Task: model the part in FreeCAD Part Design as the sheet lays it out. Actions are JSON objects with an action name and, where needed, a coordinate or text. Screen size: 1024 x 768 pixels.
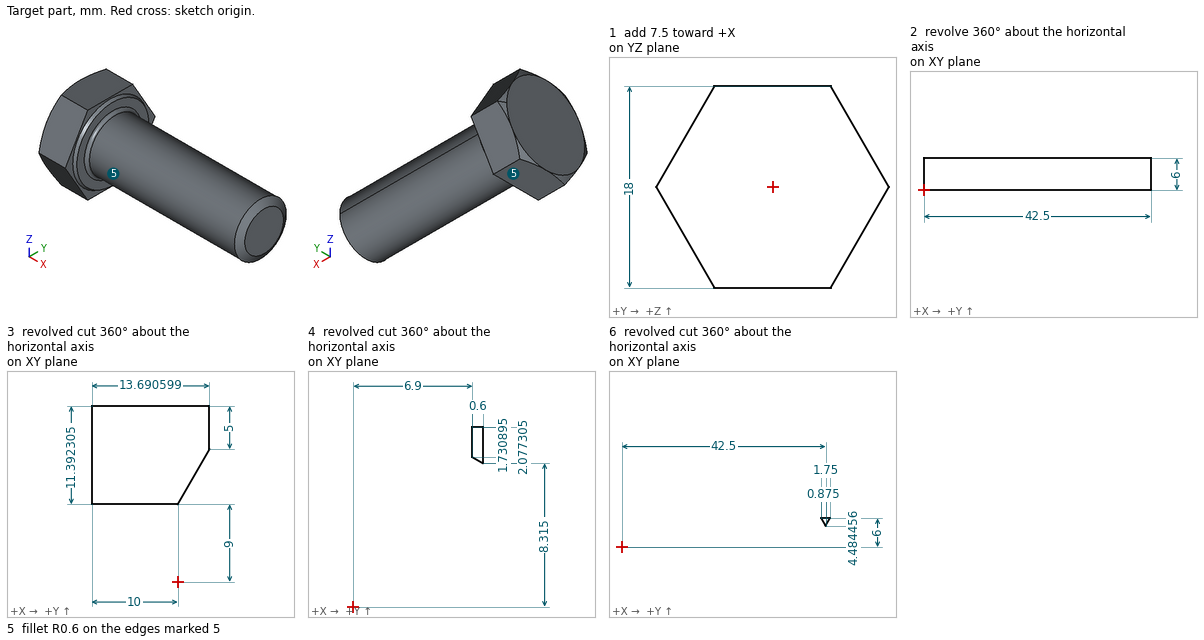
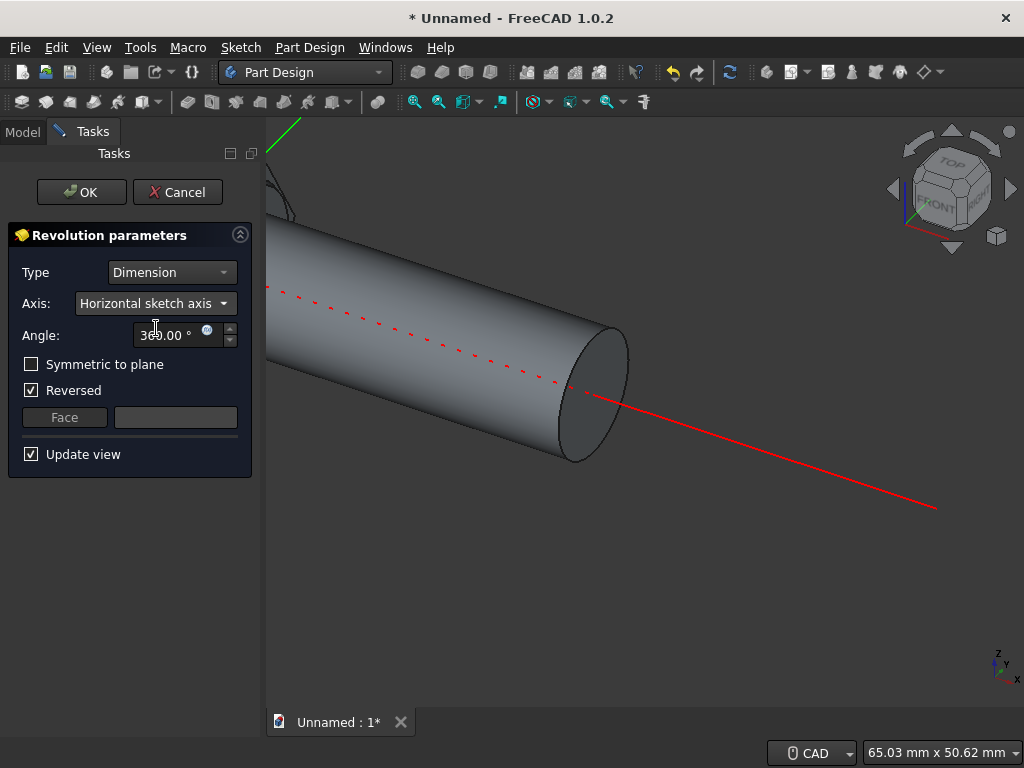
{"action": "left_click", "coordinate": [82, 192]}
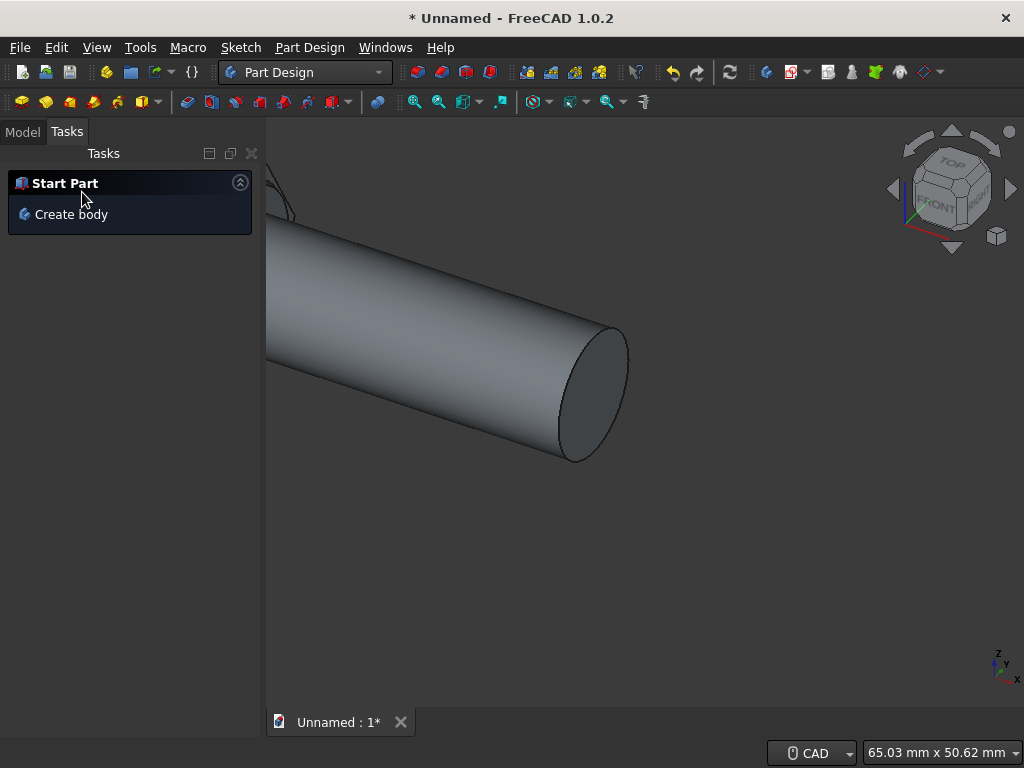
{"action": "left_click", "coordinate": [416, 102]}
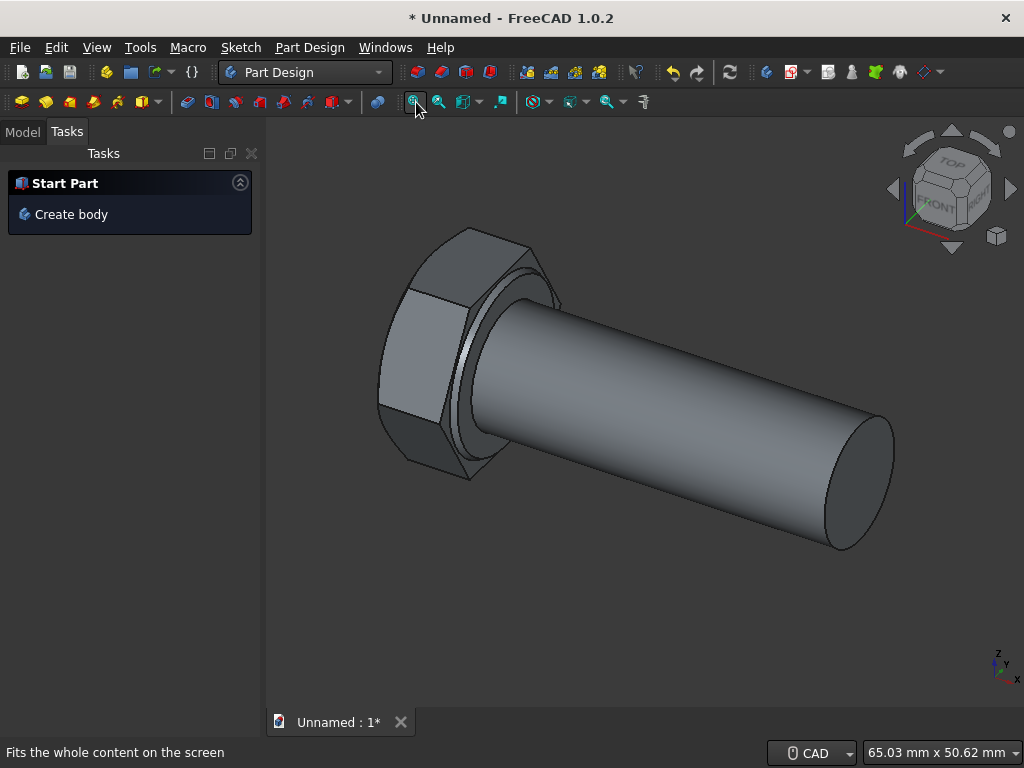
{"action": "key", "text": "0"}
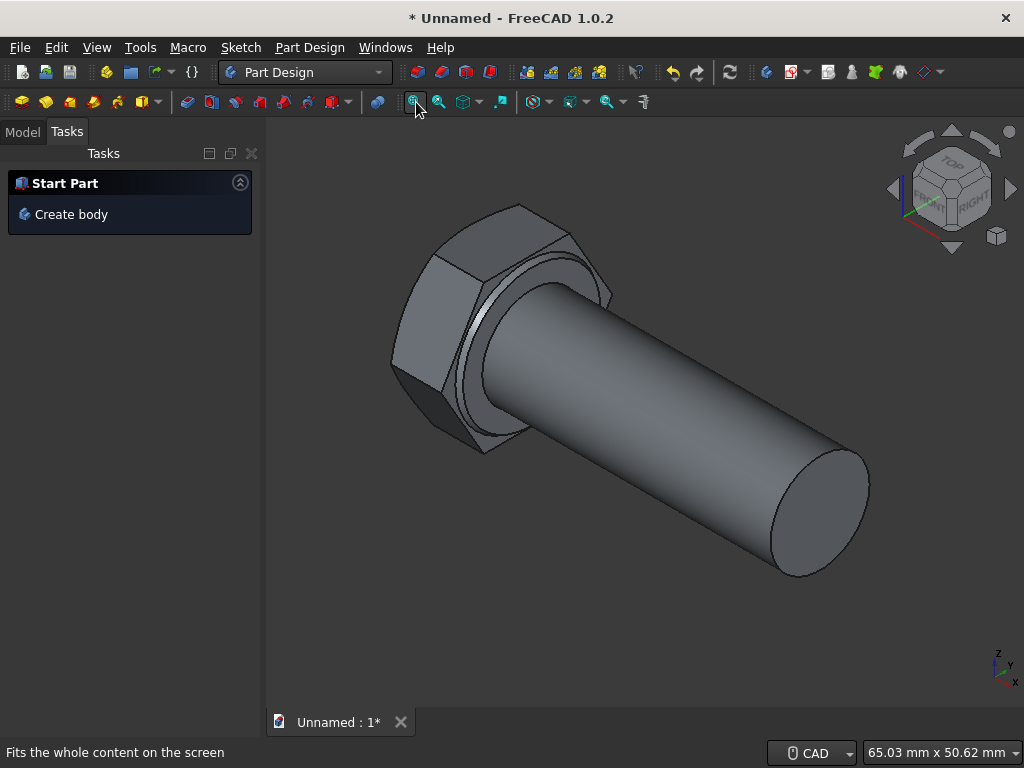
{"action": "key", "text": "2"}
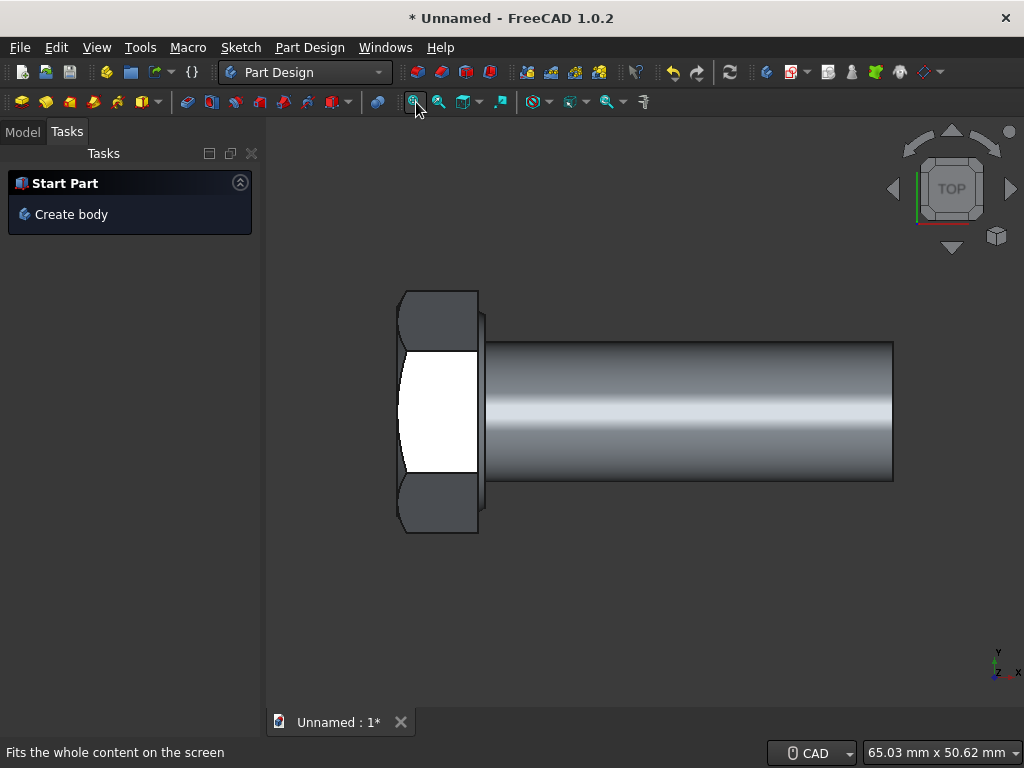
{"action": "key", "text": "1"}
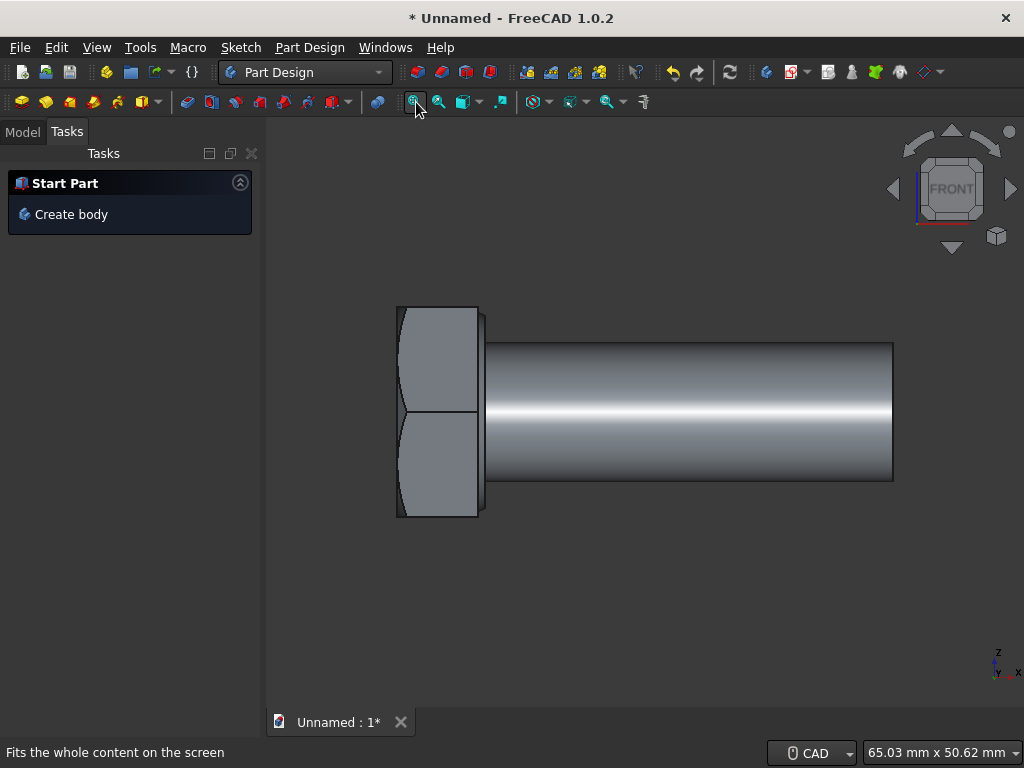
{"action": "key", "text": "3"}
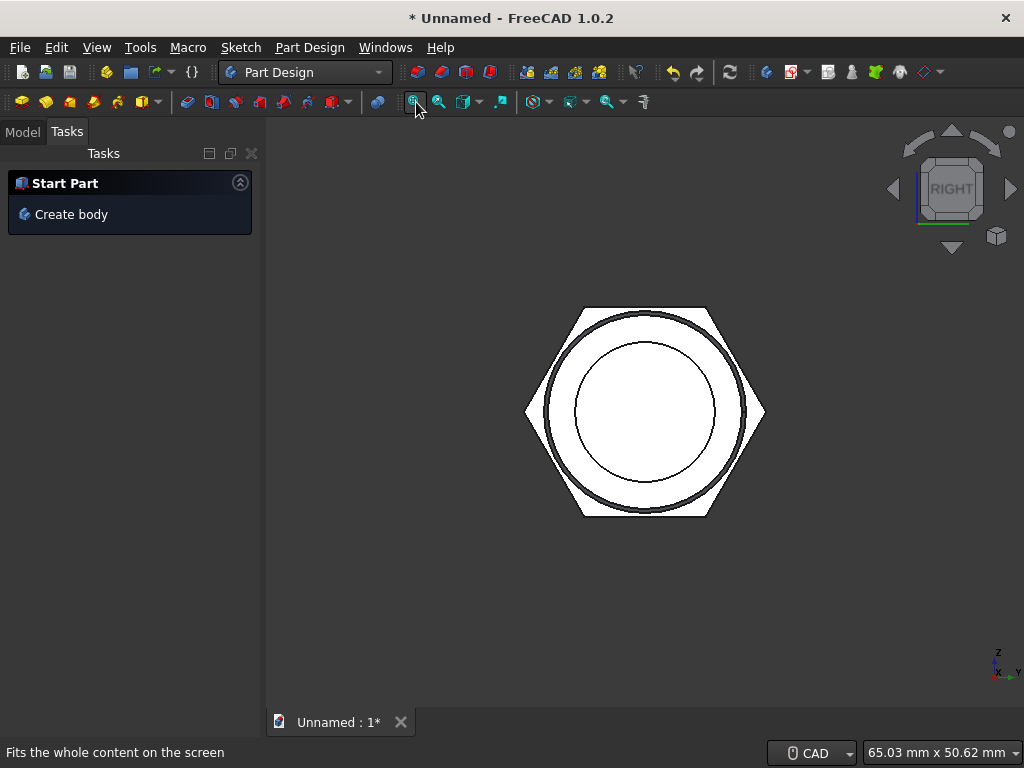
{"action": "left_click", "coordinate": [416, 102]}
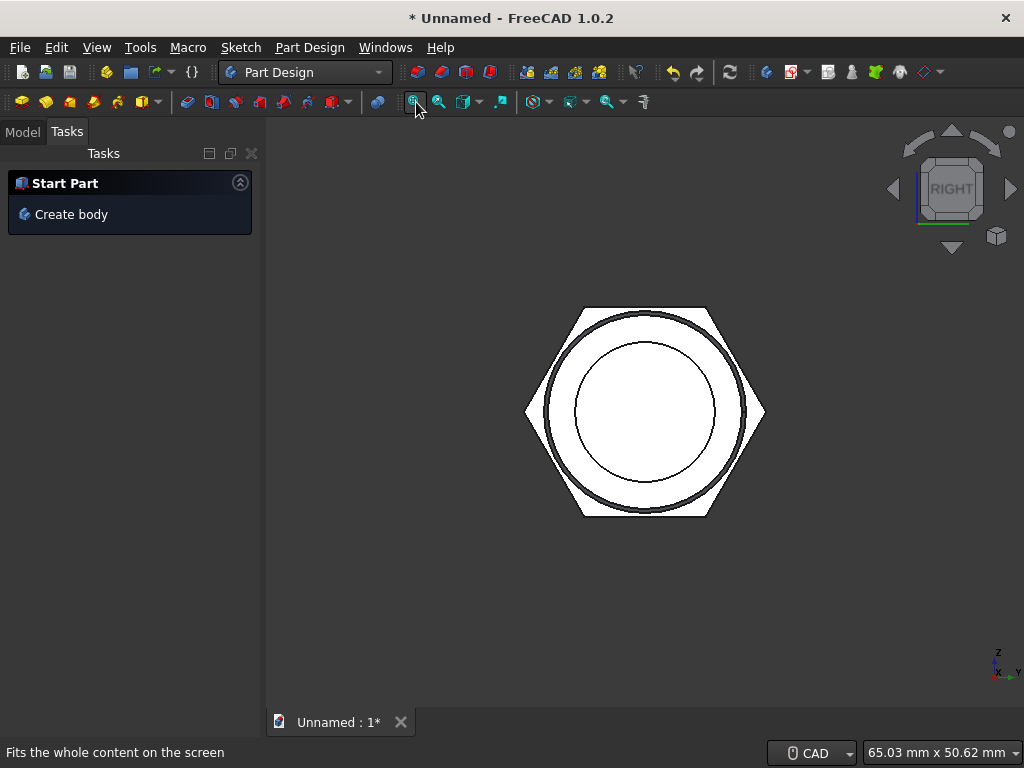
{"action": "key", "text": "5"}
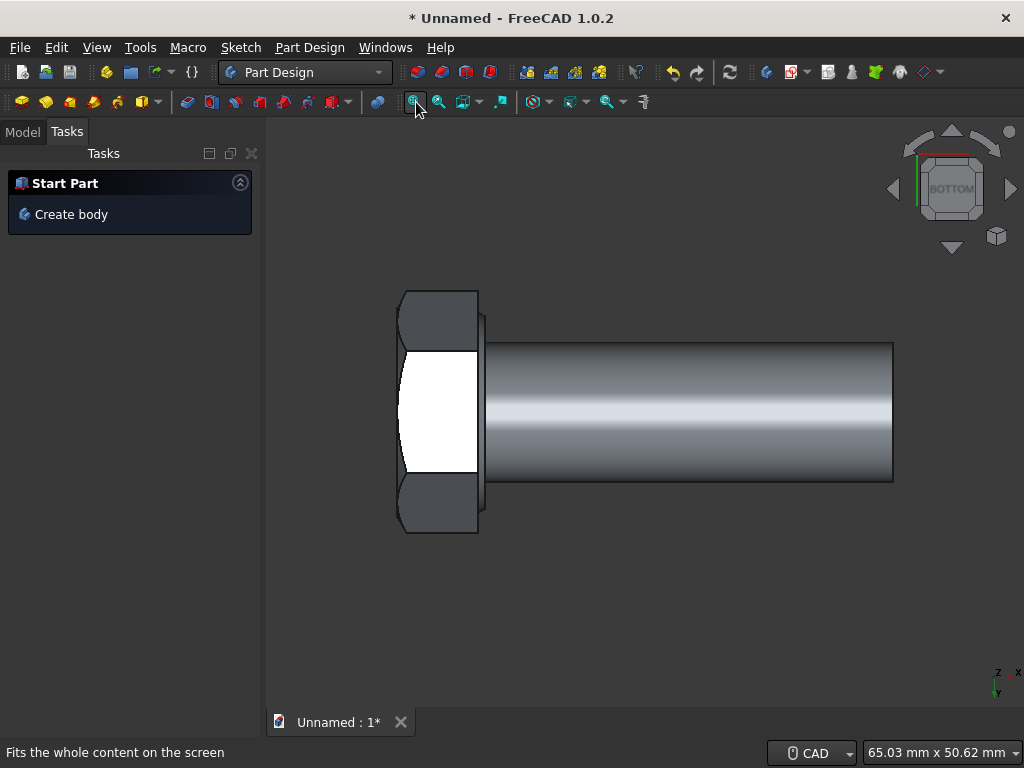
{"action": "key", "text": "4"}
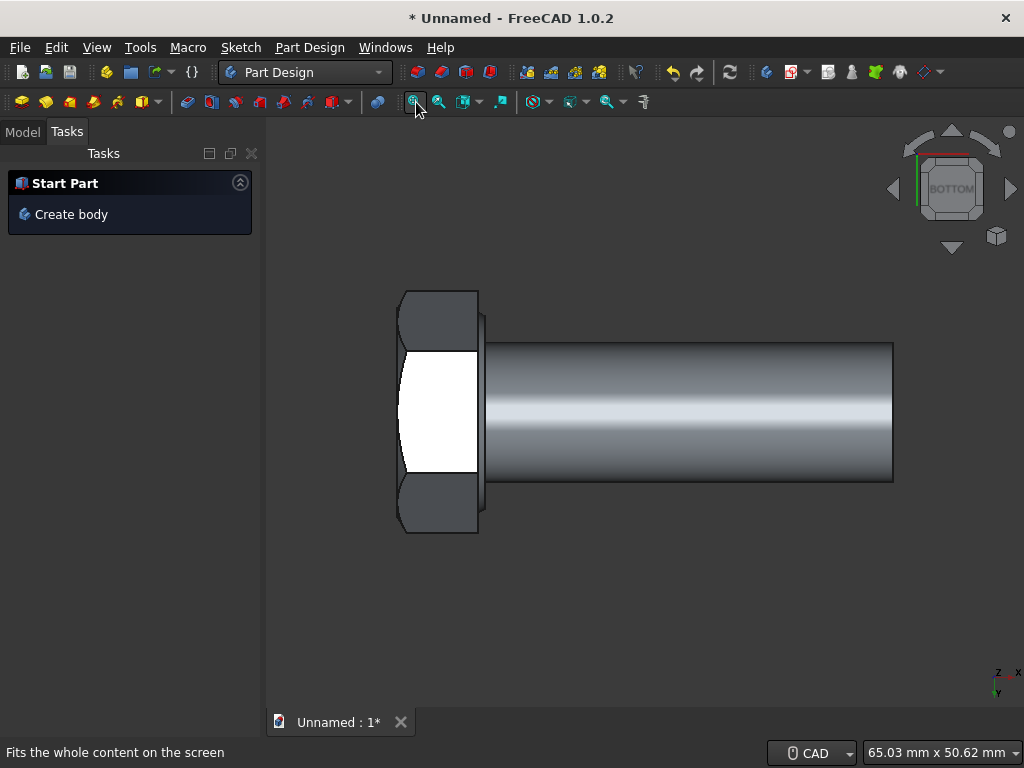
{"action": "key", "text": "6"}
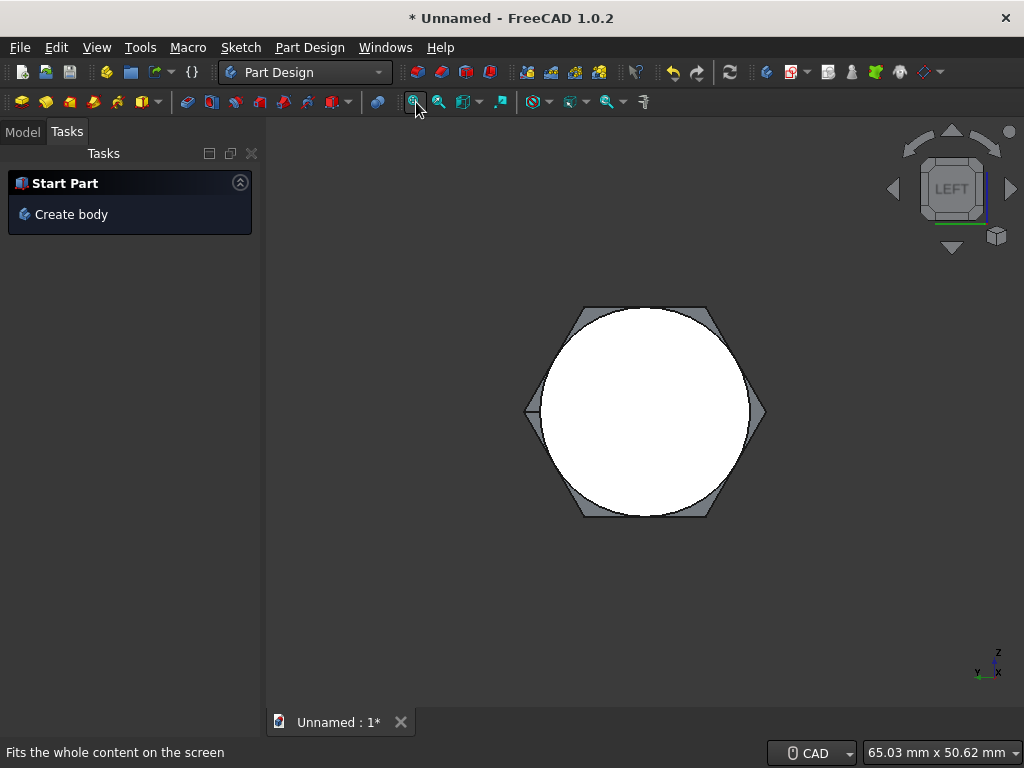
{"action": "left_click", "coordinate": [416, 102]}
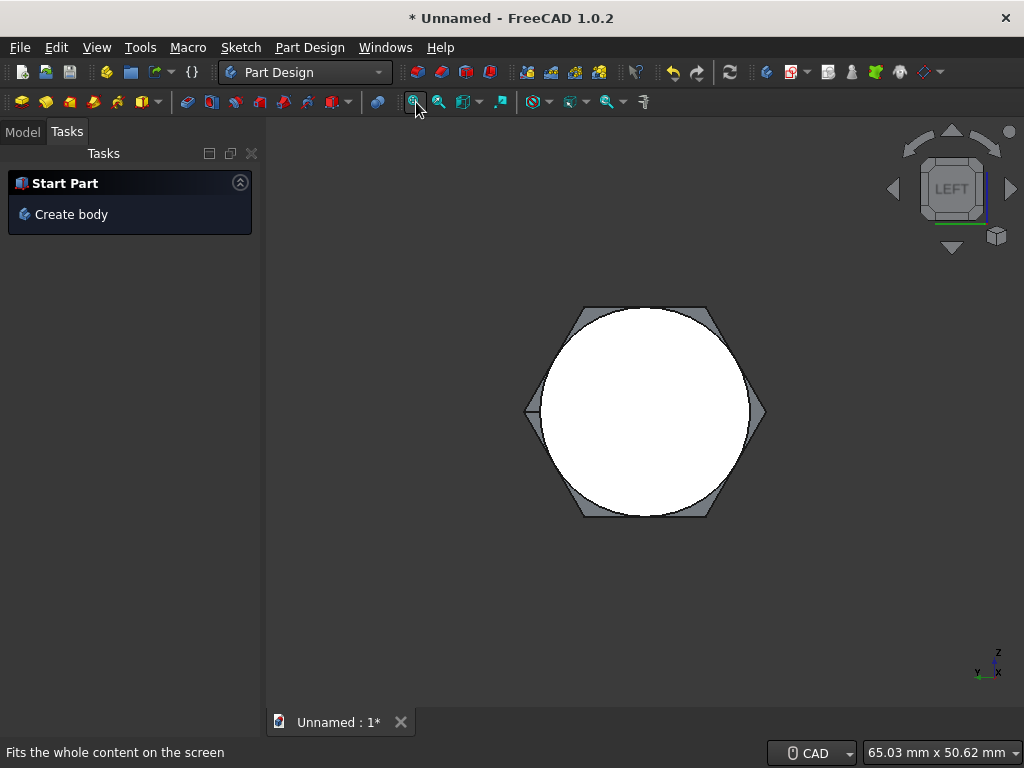
{"action": "key", "text": "v 3"}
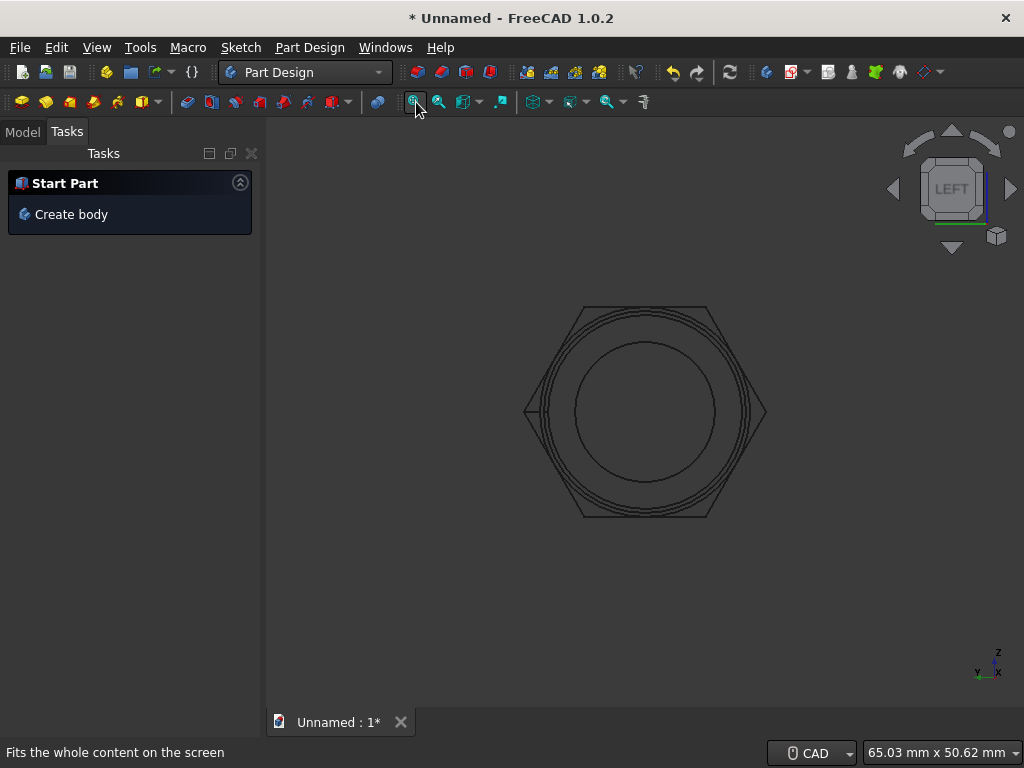
{"action": "key", "text": "0"}